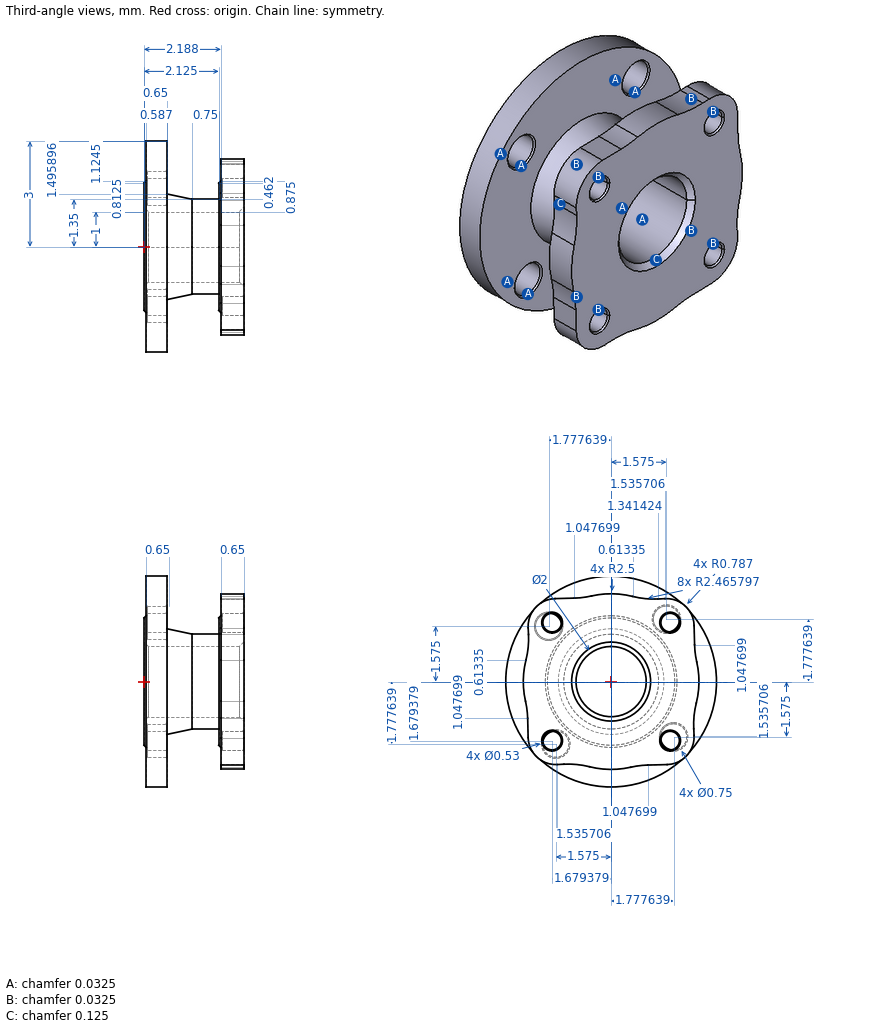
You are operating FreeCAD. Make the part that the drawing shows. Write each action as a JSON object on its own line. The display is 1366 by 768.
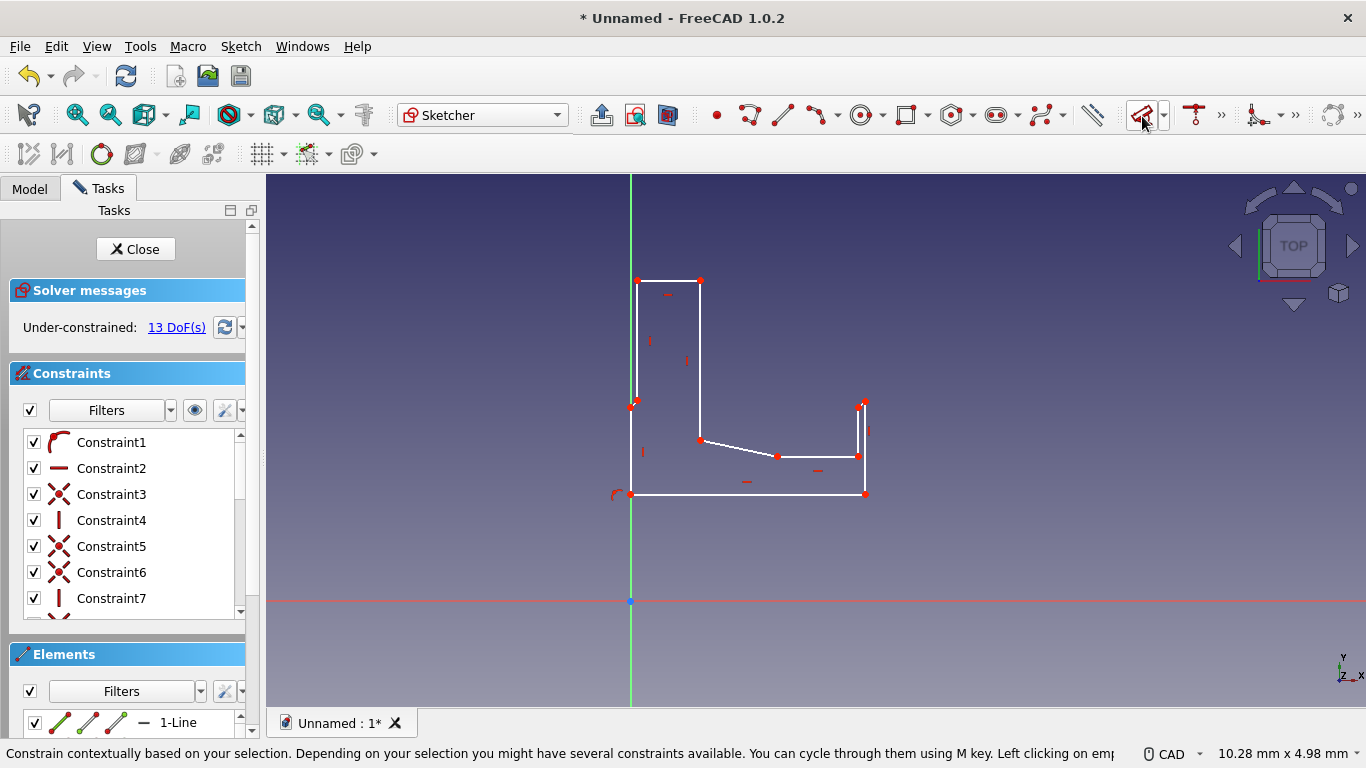
{"action": "left_click", "coordinate": [631, 495]}
{"action": "left_click", "coordinate": [597, 548]}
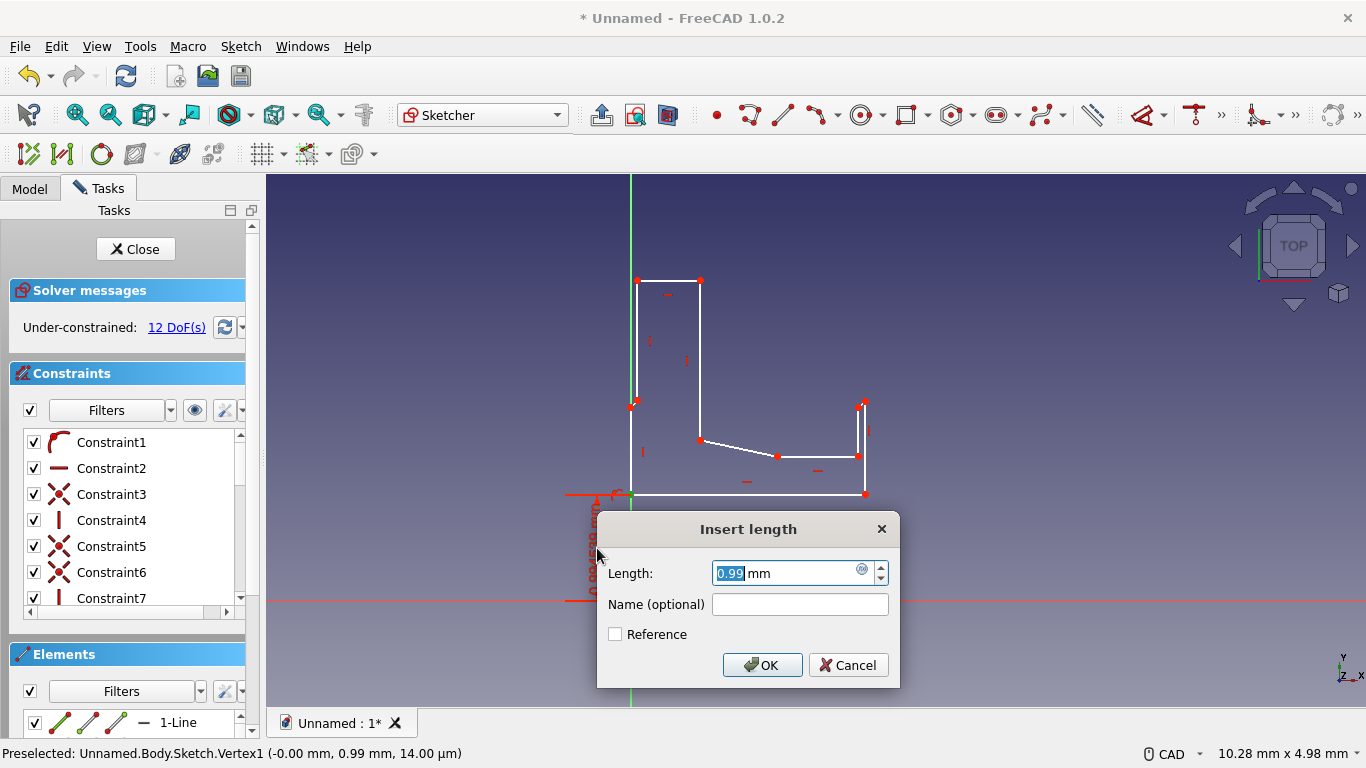
{"action": "type", "text": "1"}
{"action": "key", "text": "Return"}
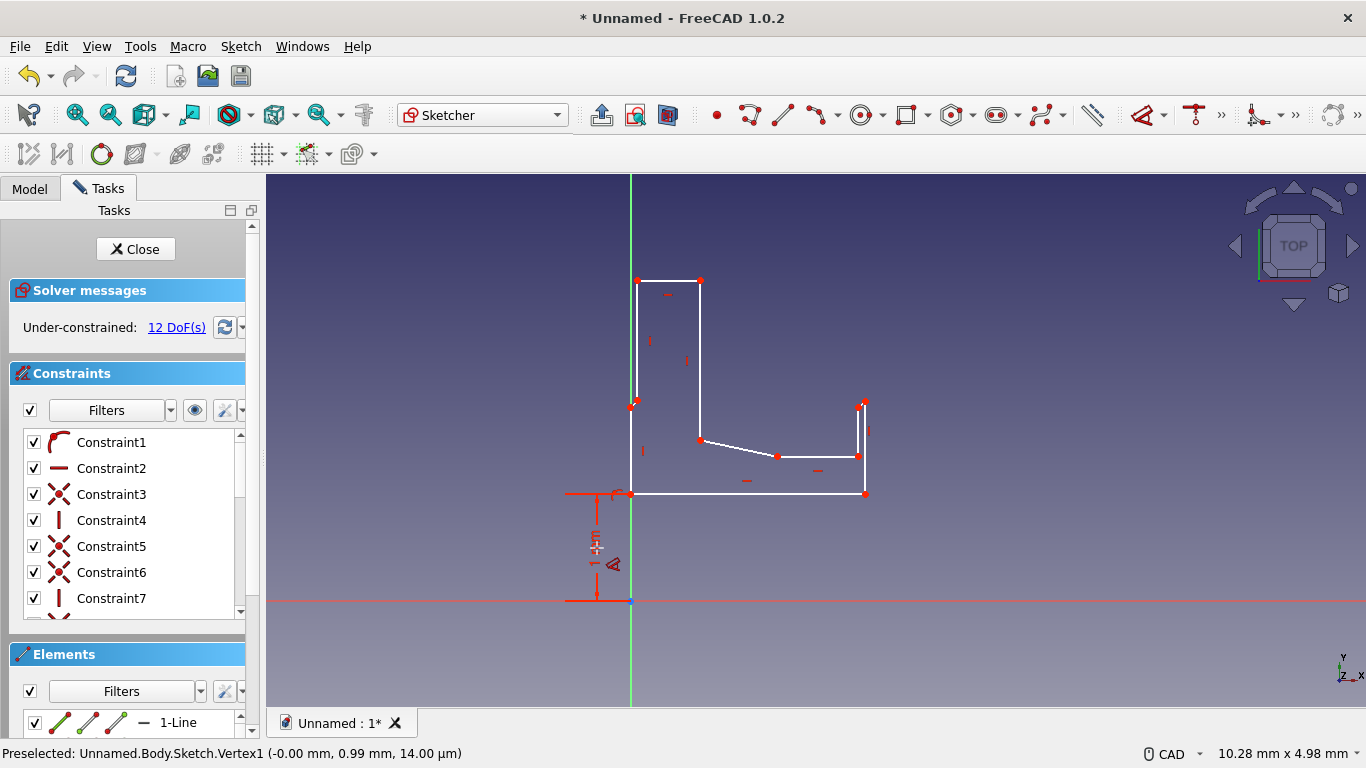
{"action": "left_click", "coordinate": [700, 281]}
{"action": "left_click", "coordinate": [597, 441]}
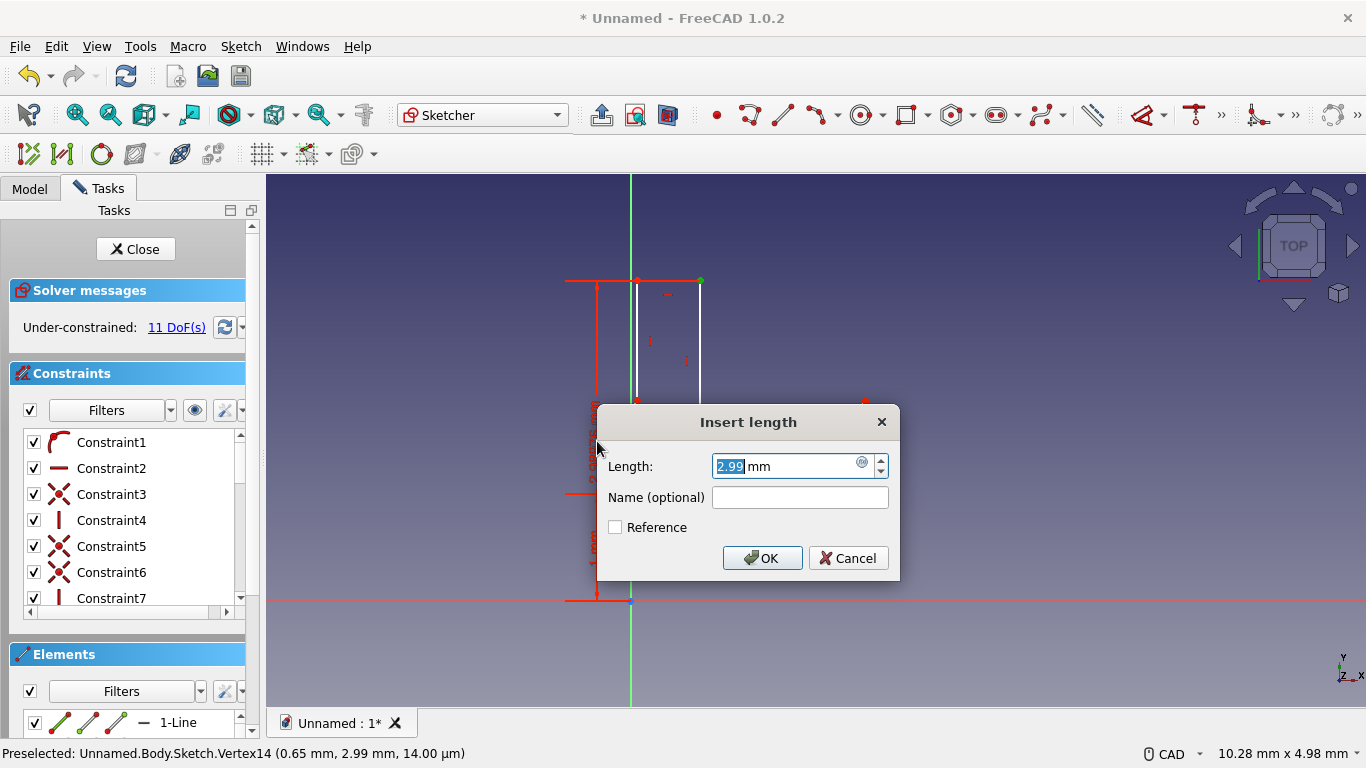
{"action": "type", "text": "3"}
{"action": "key", "text": "Return"}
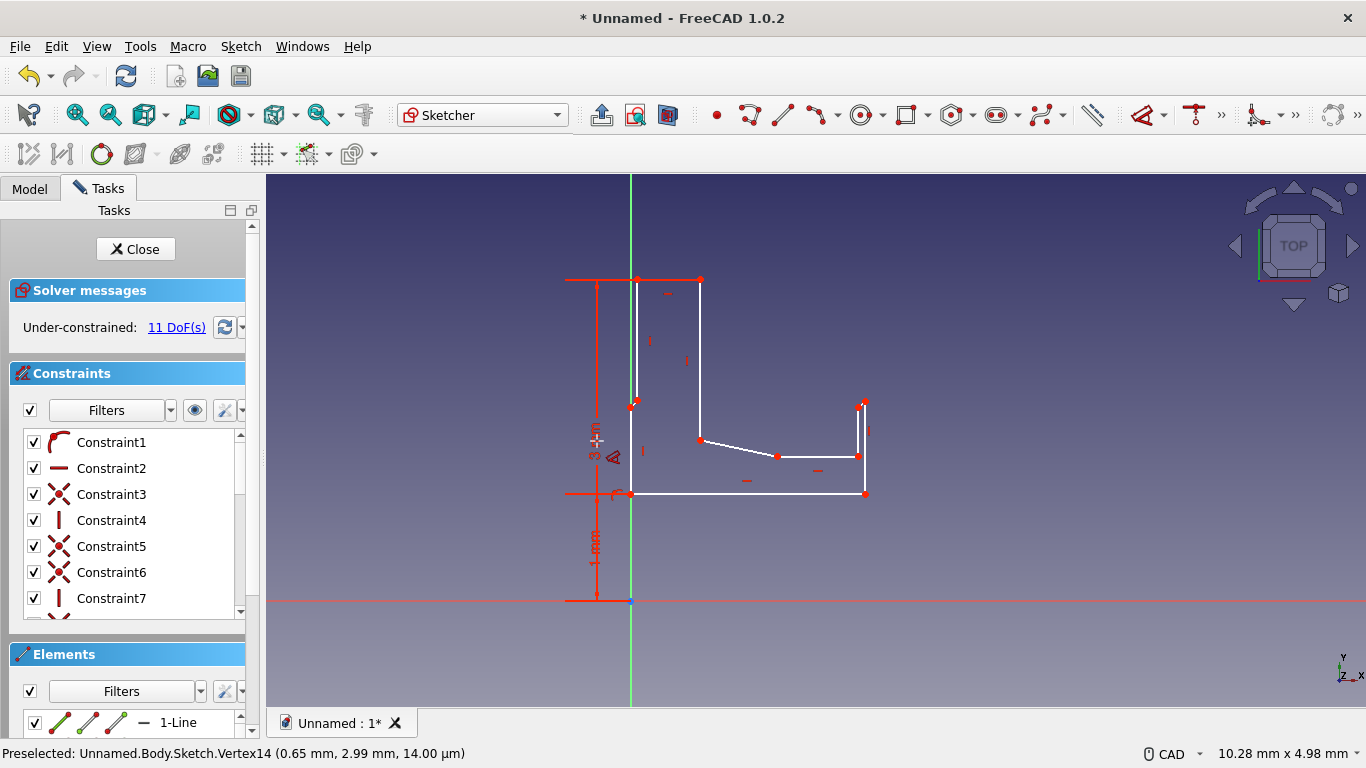
{"action": "left_click", "coordinate": [834, 457]}
{"action": "left_click", "coordinate": [818, 423]}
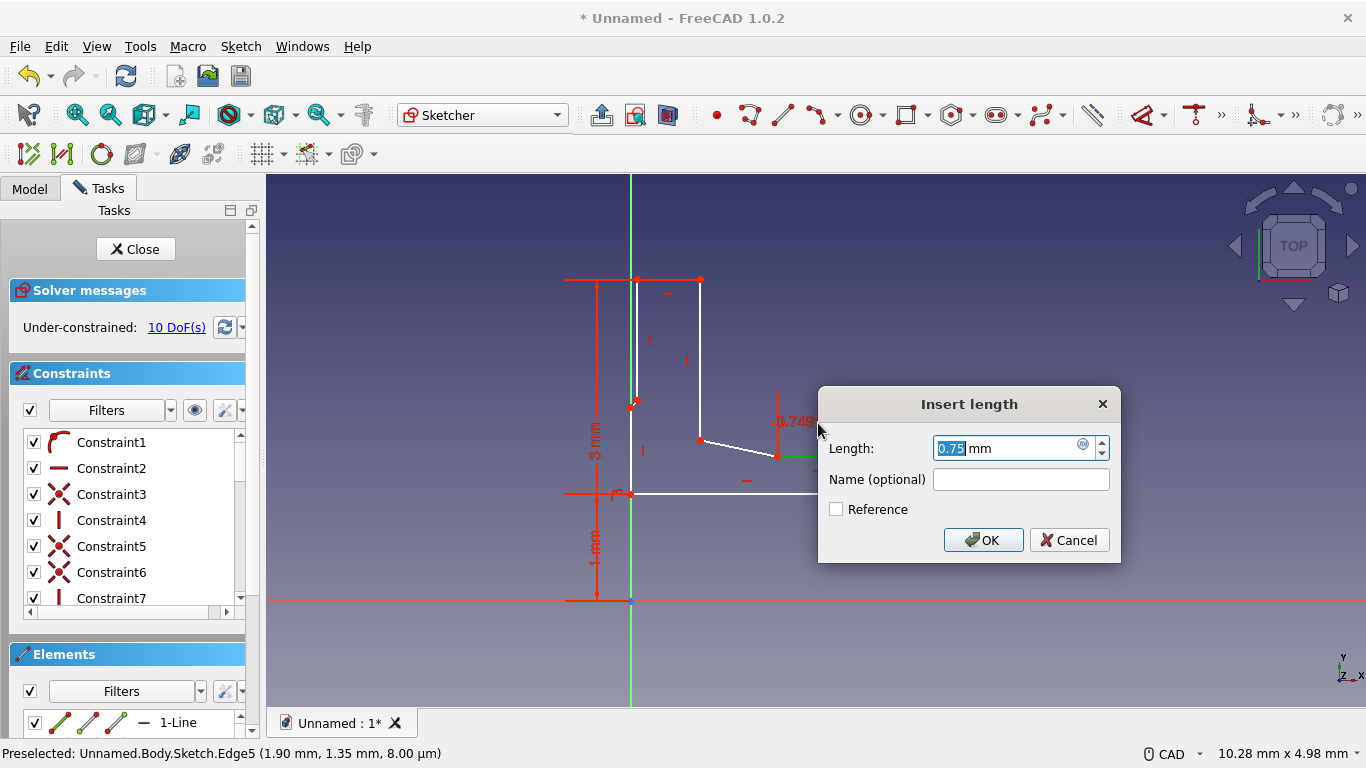
{"action": "type", "text": "0.75"}
{"action": "key", "text": "Return"}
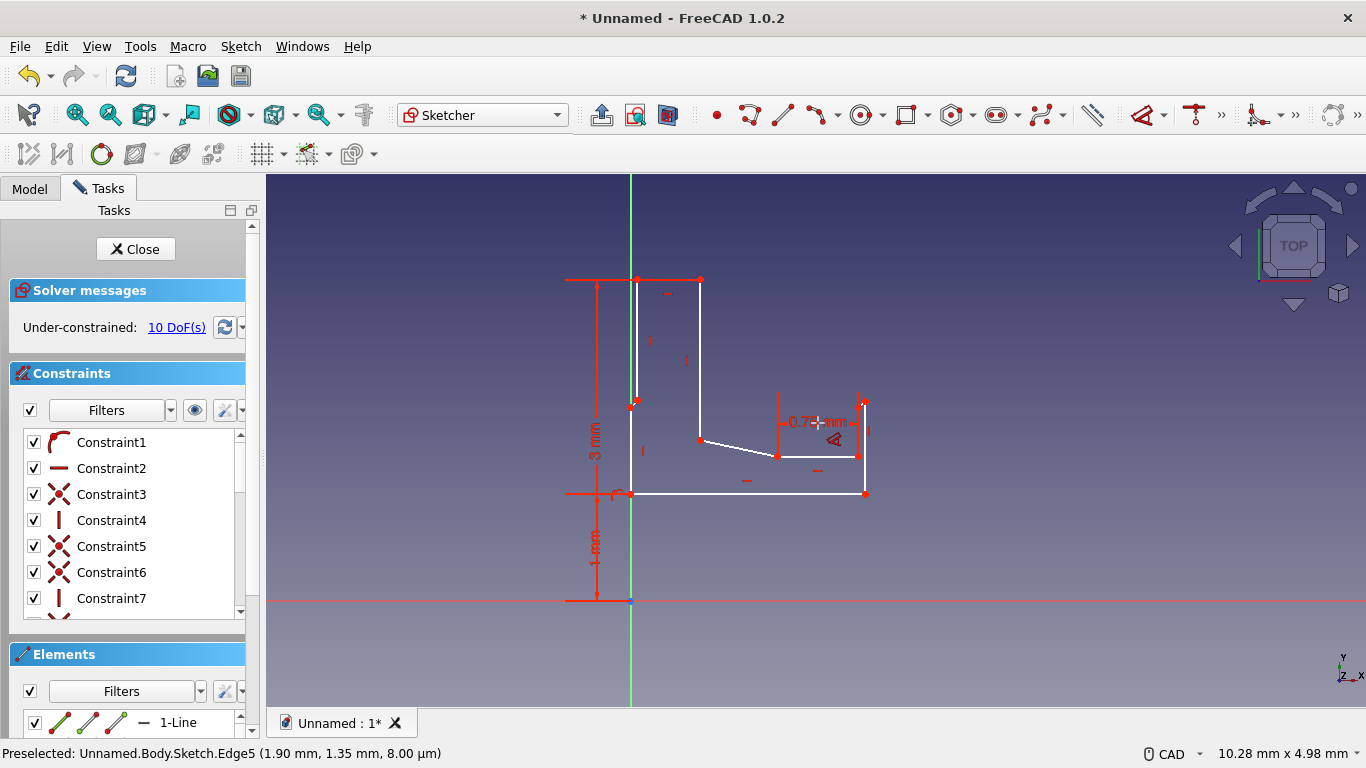
{"action": "left_click", "coordinate": [701, 494]}
{"action": "left_click", "coordinate": [748, 528]}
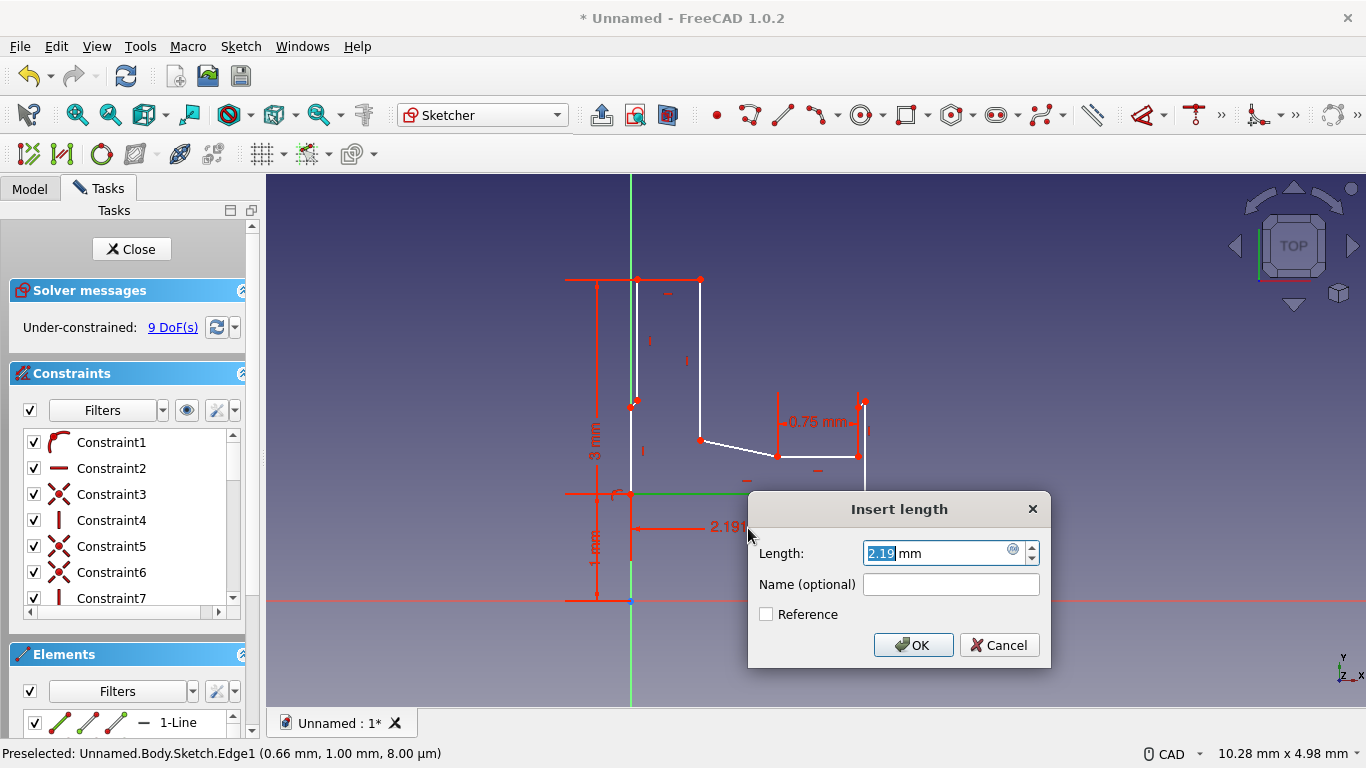
{"action": "type", "text": "2.188"}
{"action": "key", "text": "Return"}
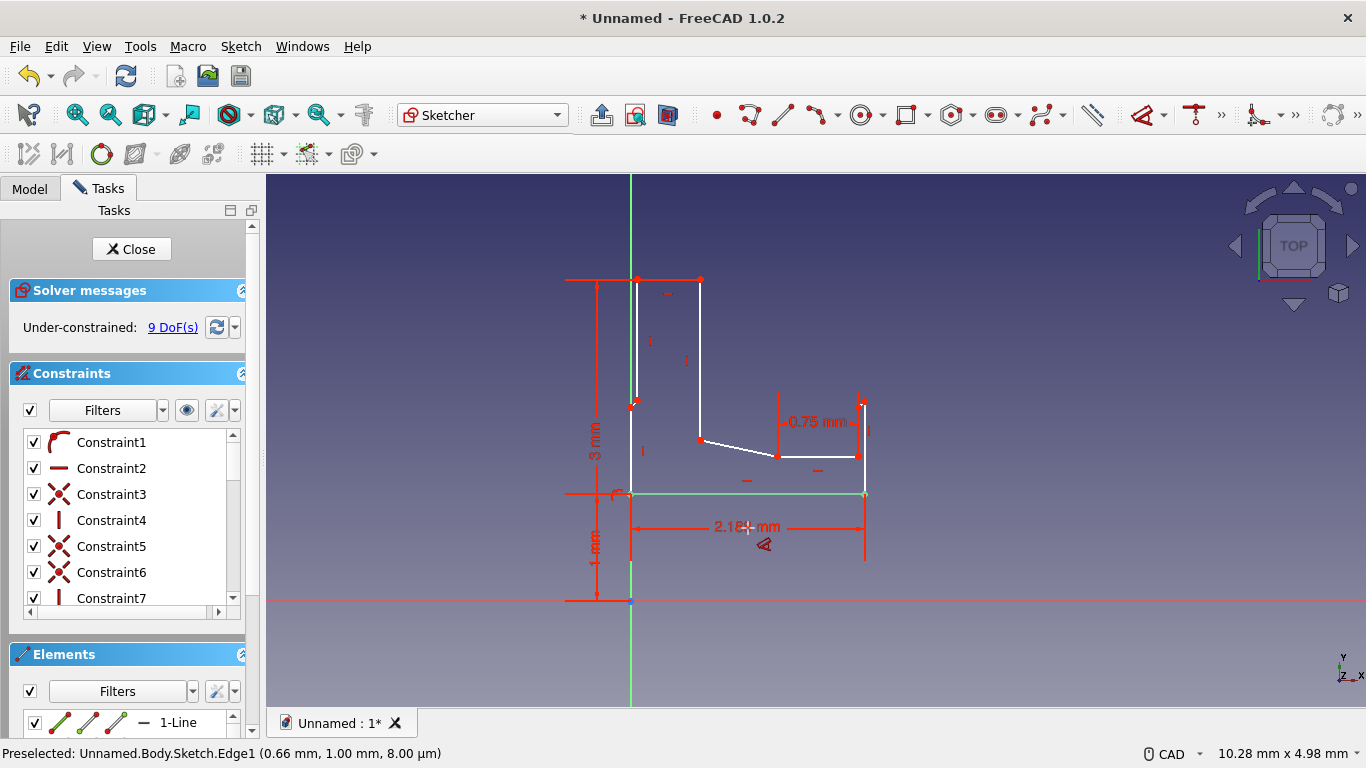
{"action": "left_click", "coordinate": [865, 466]}
{"action": "left_click", "coordinate": [899, 448]}